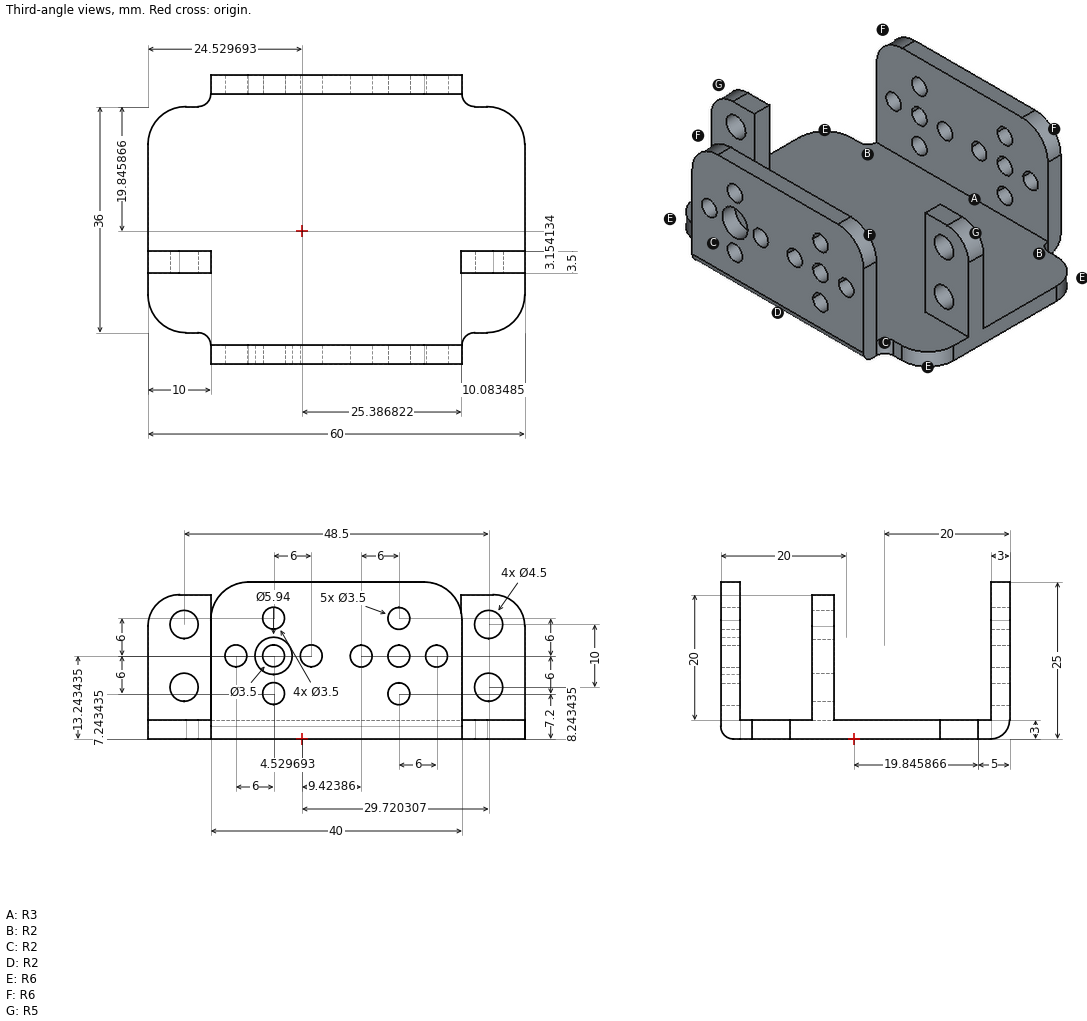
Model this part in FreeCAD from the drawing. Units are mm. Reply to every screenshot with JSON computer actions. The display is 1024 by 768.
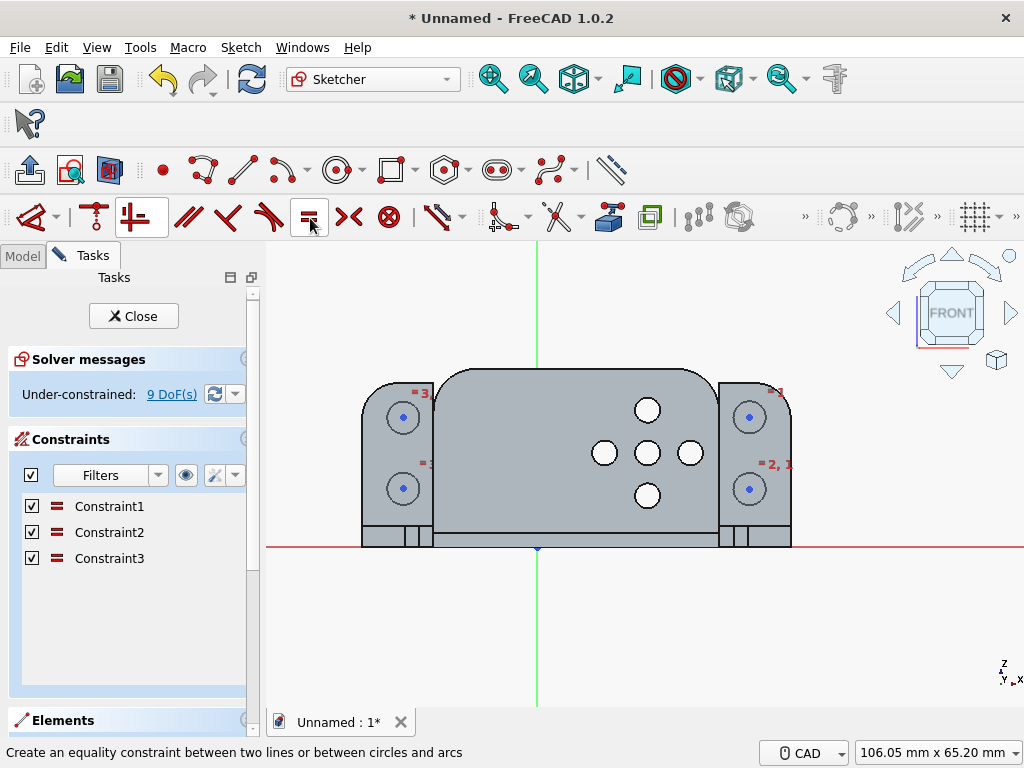
{"action": "left_click", "coordinate": [750, 417]}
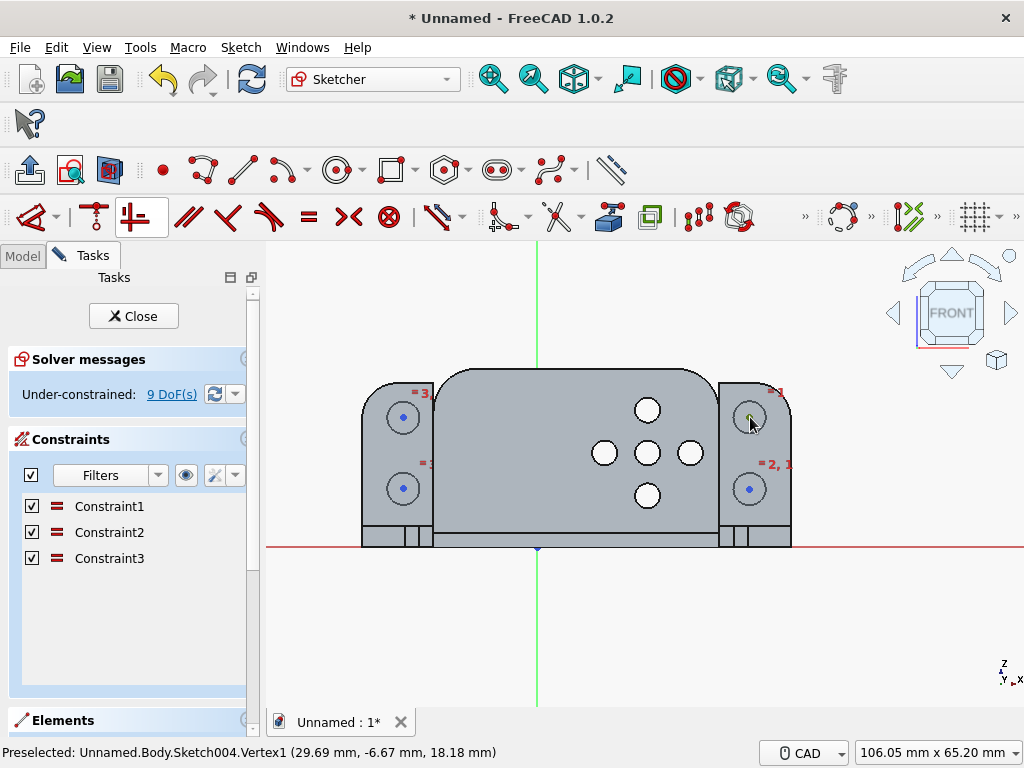
{"action": "left_click", "coordinate": [750, 489]}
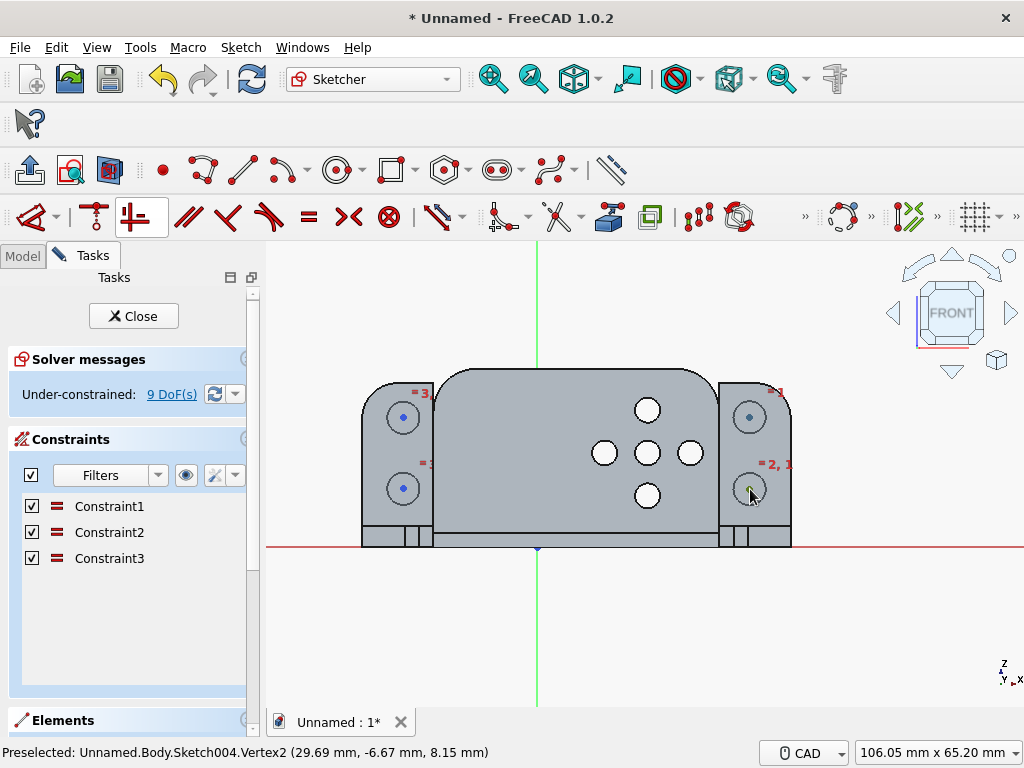
{"action": "left_click", "coordinate": [162, 218]}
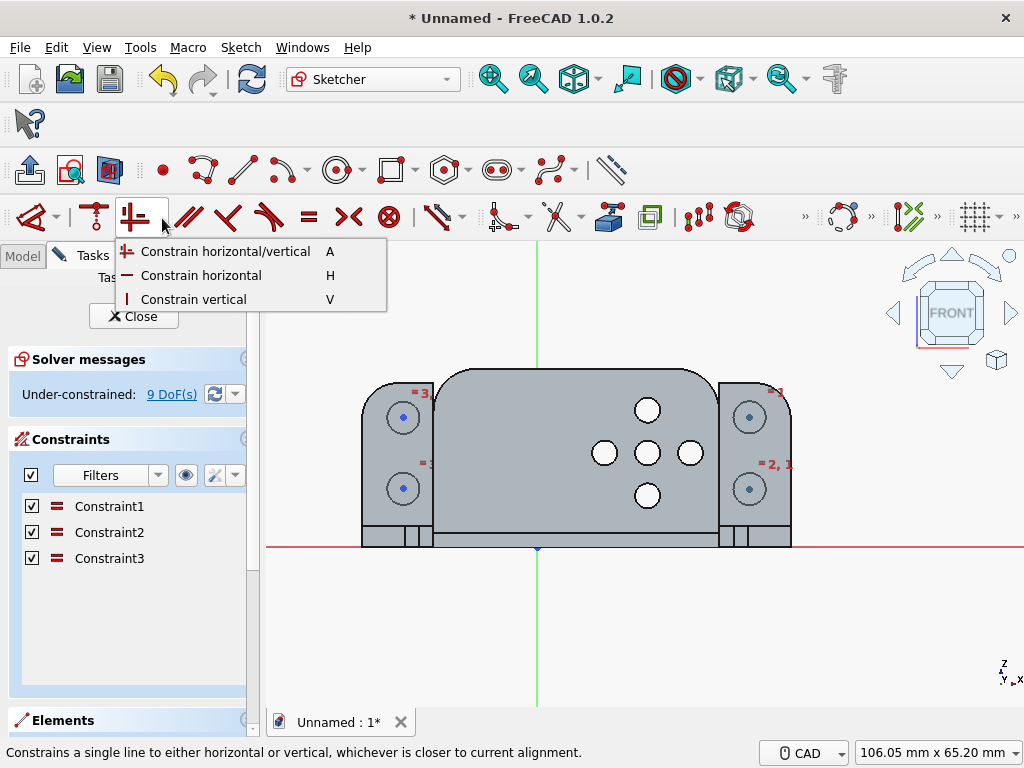
{"action": "left_click", "coordinate": [251, 299]}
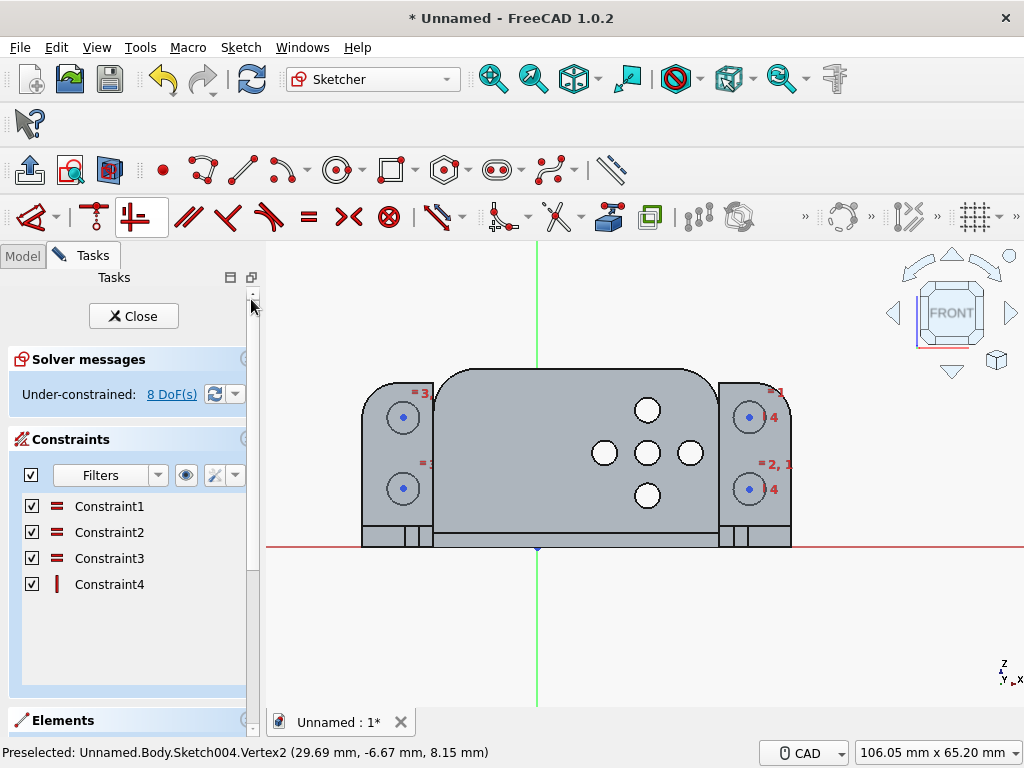
{"action": "left_click", "coordinate": [750, 417]}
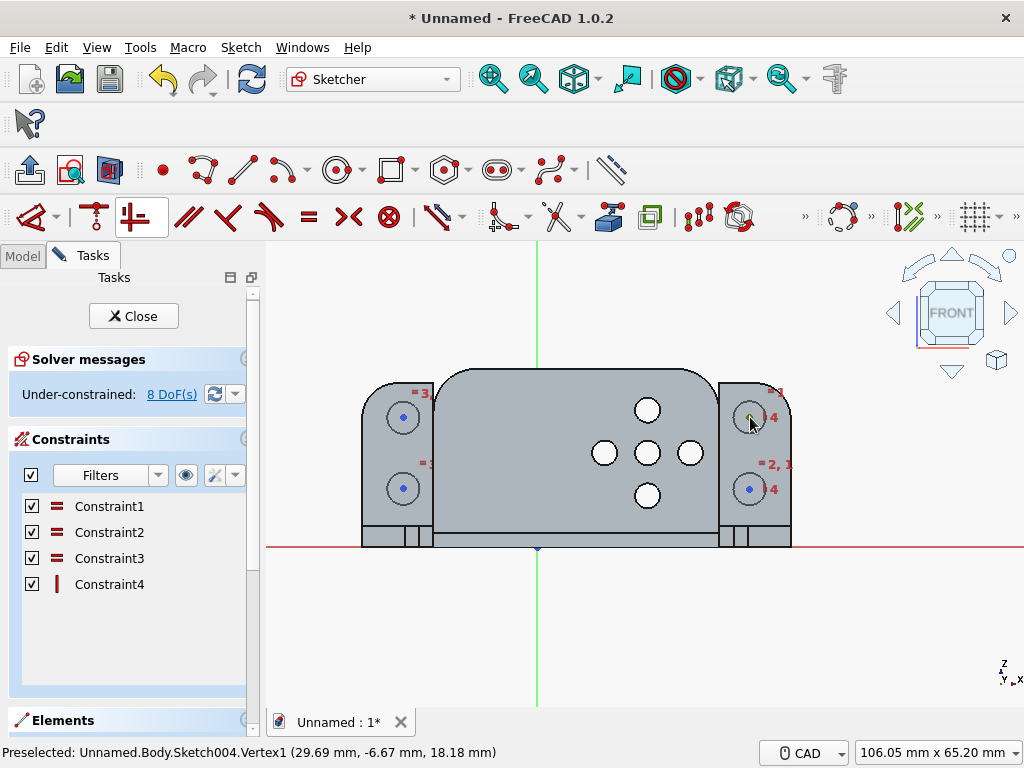
{"action": "left_click", "coordinate": [403, 418]}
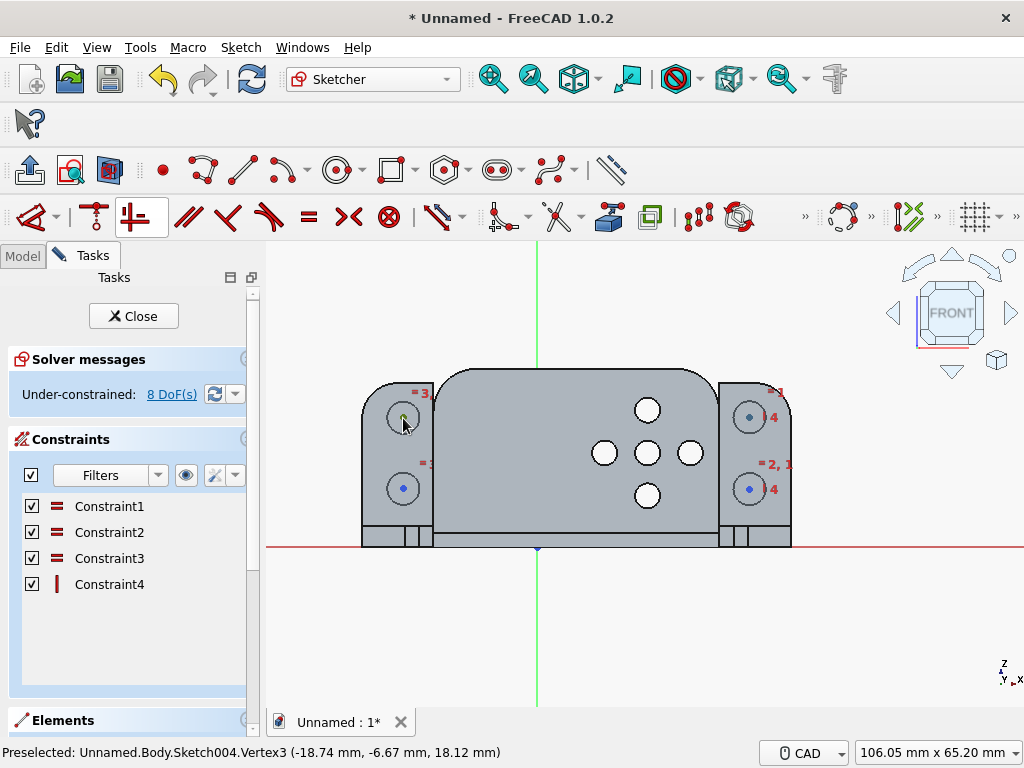
{"action": "left_click", "coordinate": [162, 218]}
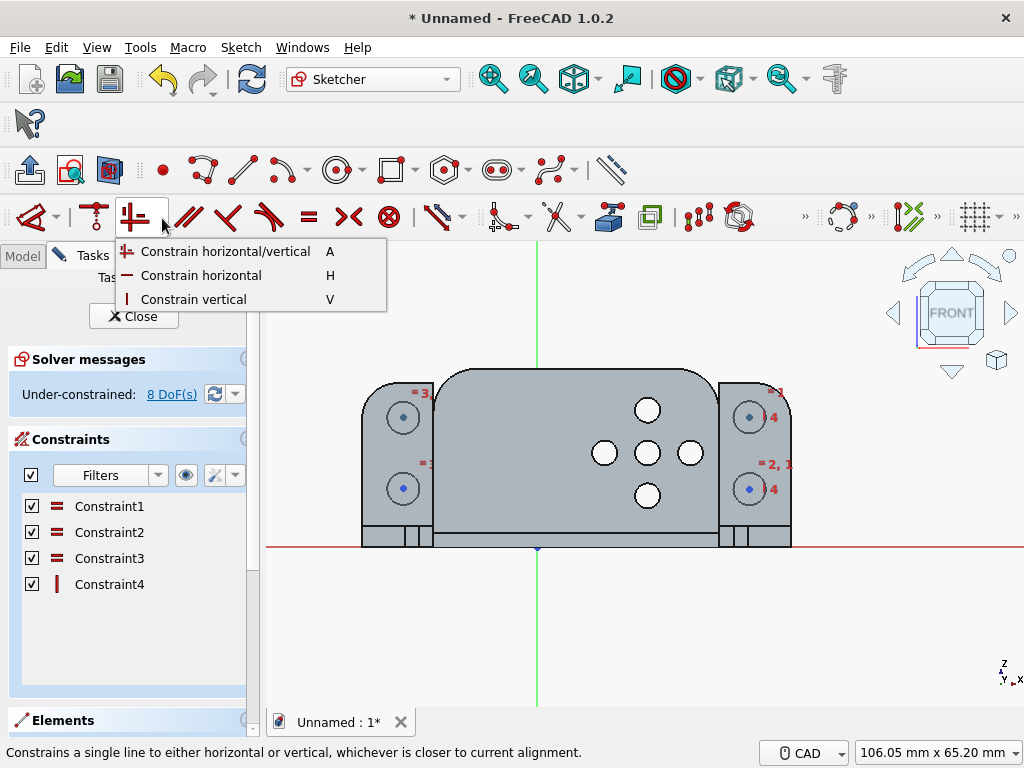
{"action": "left_click", "coordinate": [251, 275]}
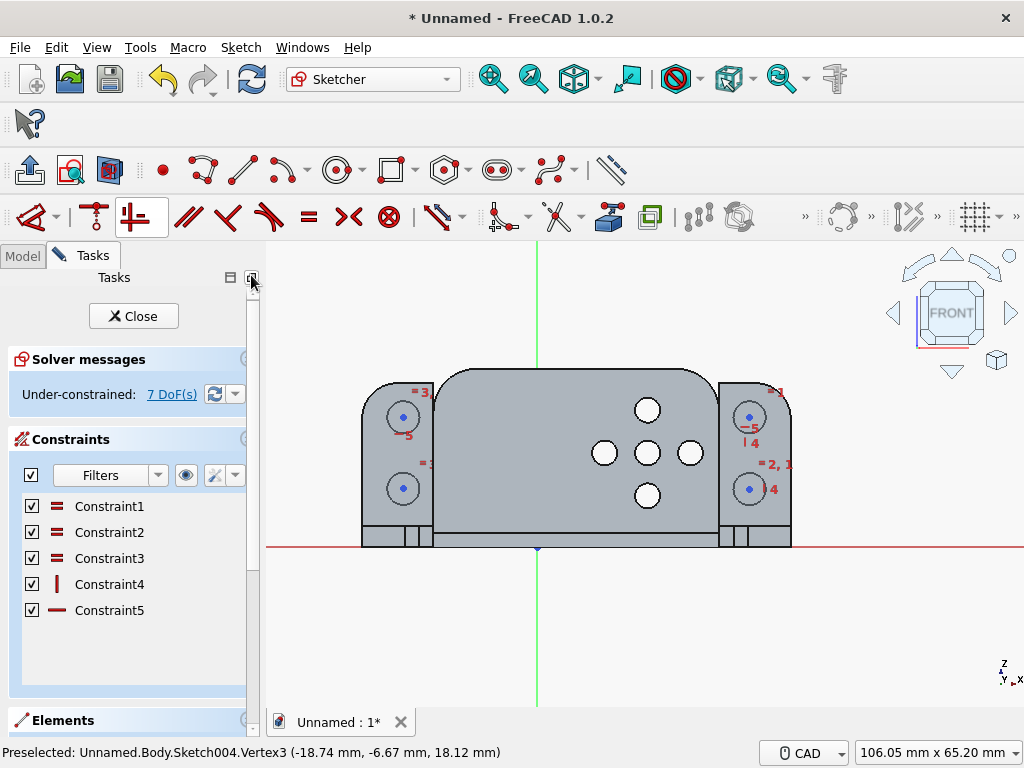
{"action": "left_click", "coordinate": [403, 417]}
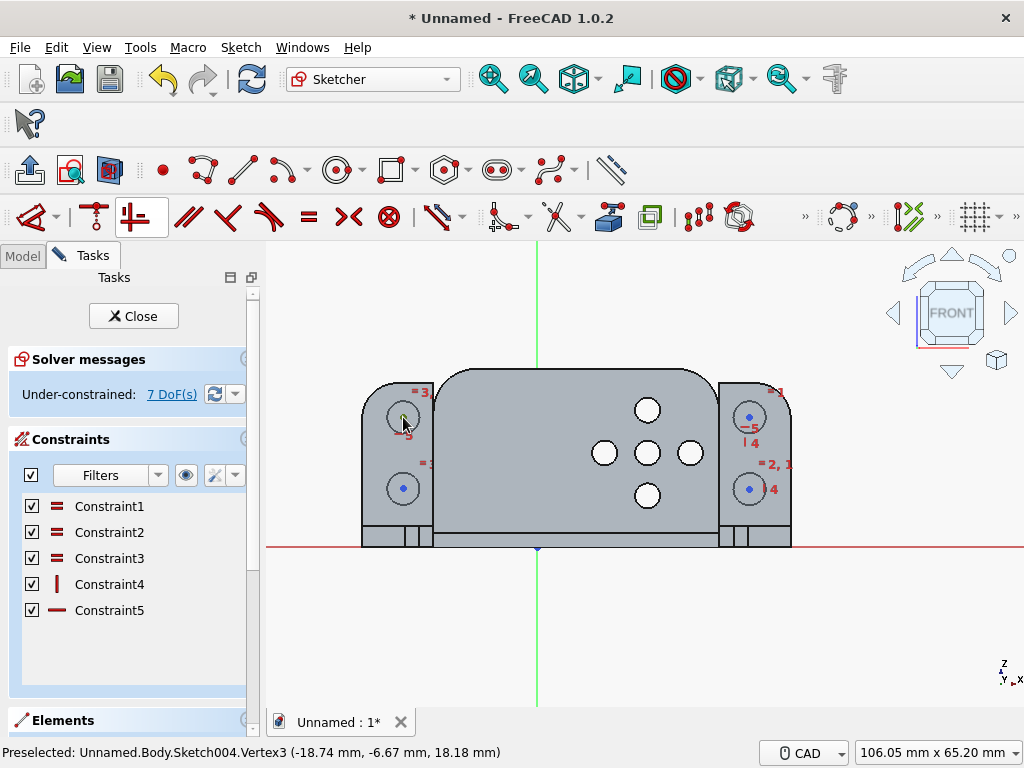
{"action": "left_click", "coordinate": [403, 489]}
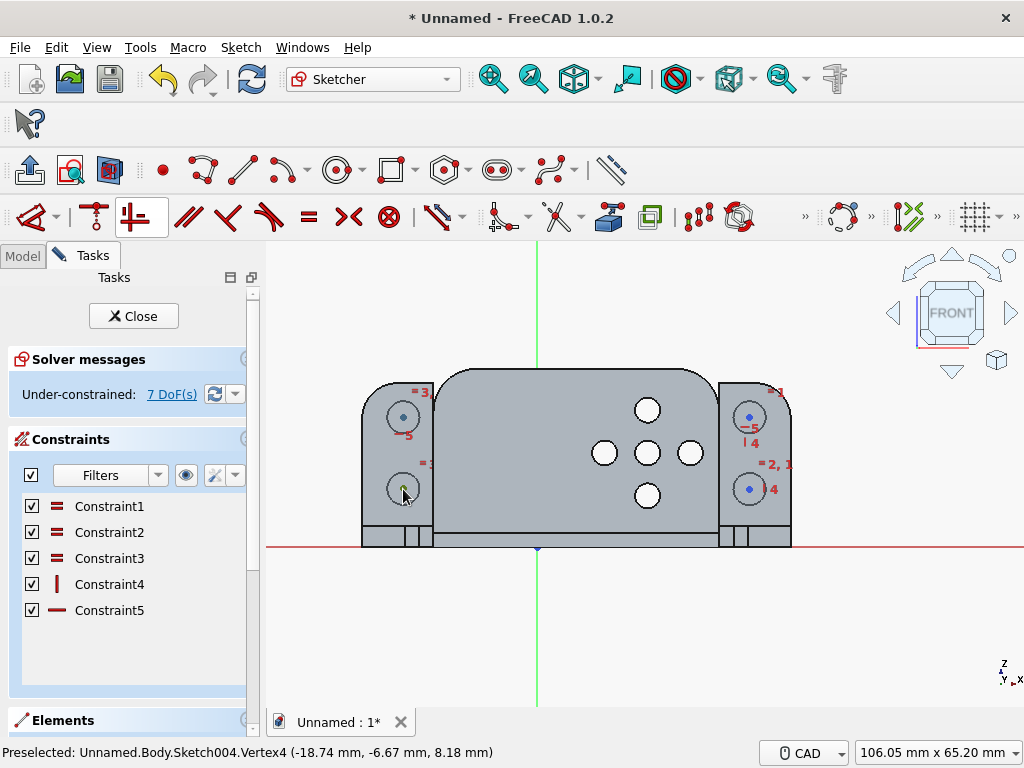
{"action": "left_click", "coordinate": [162, 218]}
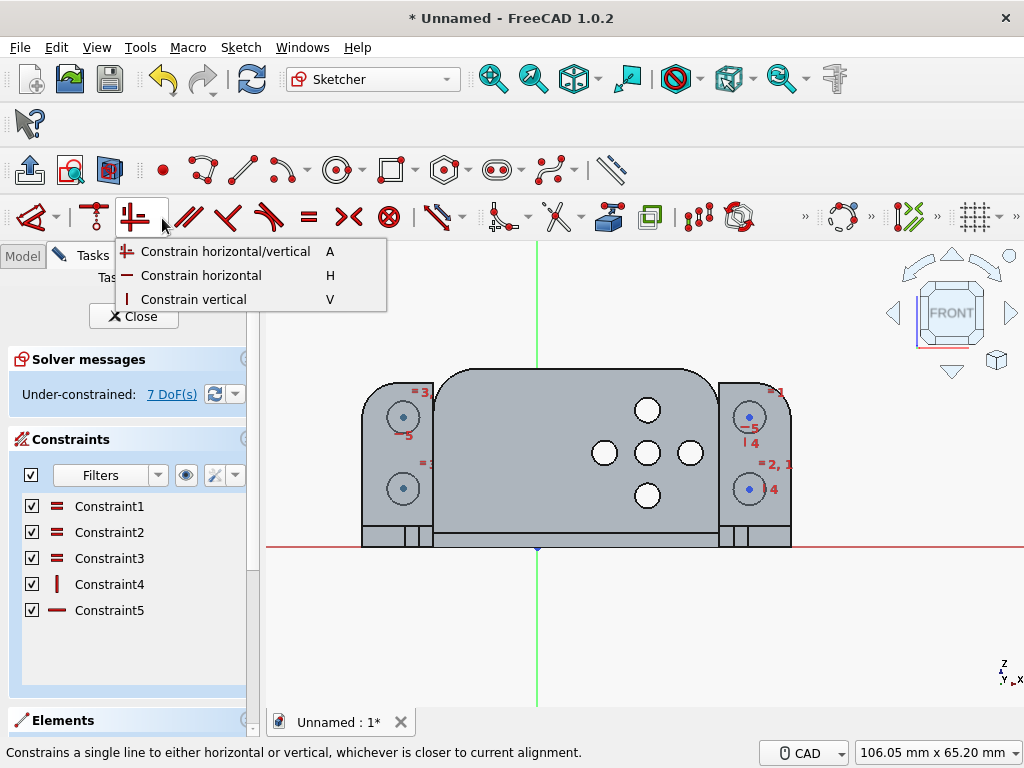
{"action": "left_click", "coordinate": [251, 299]}